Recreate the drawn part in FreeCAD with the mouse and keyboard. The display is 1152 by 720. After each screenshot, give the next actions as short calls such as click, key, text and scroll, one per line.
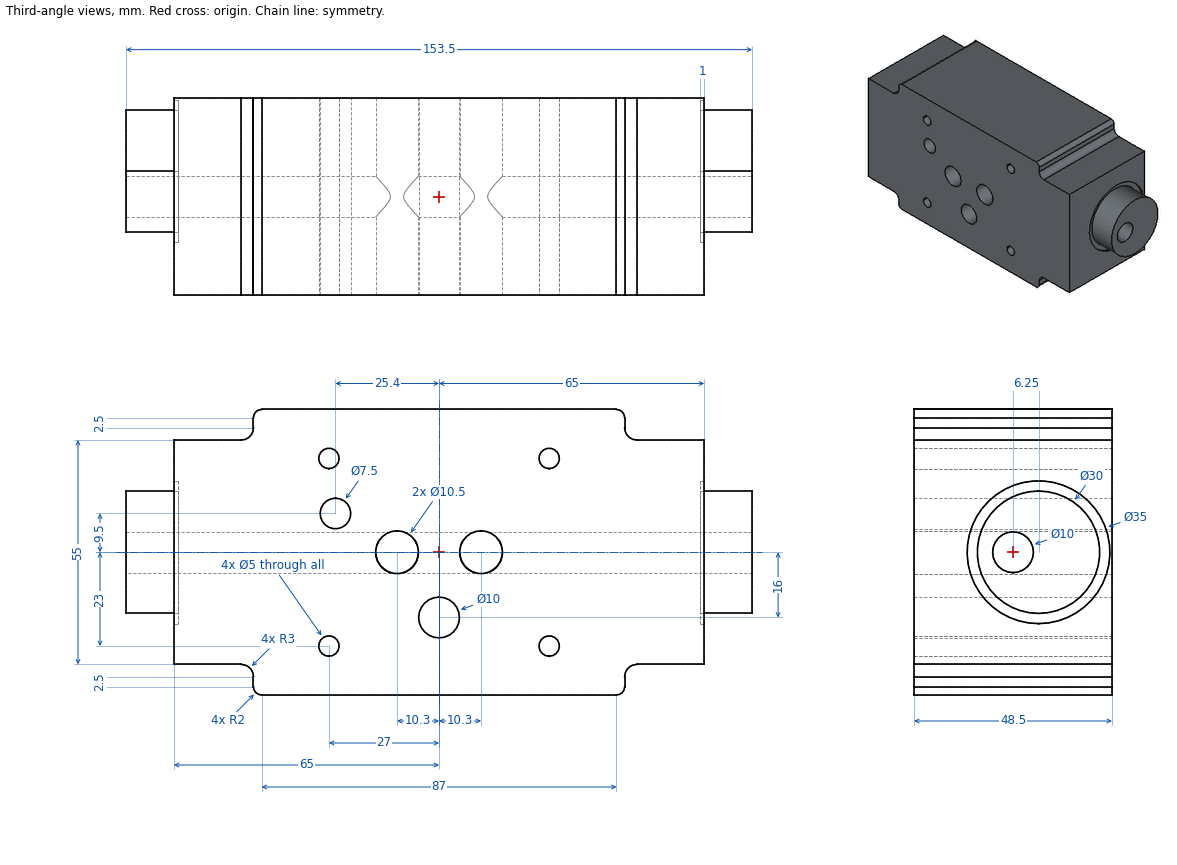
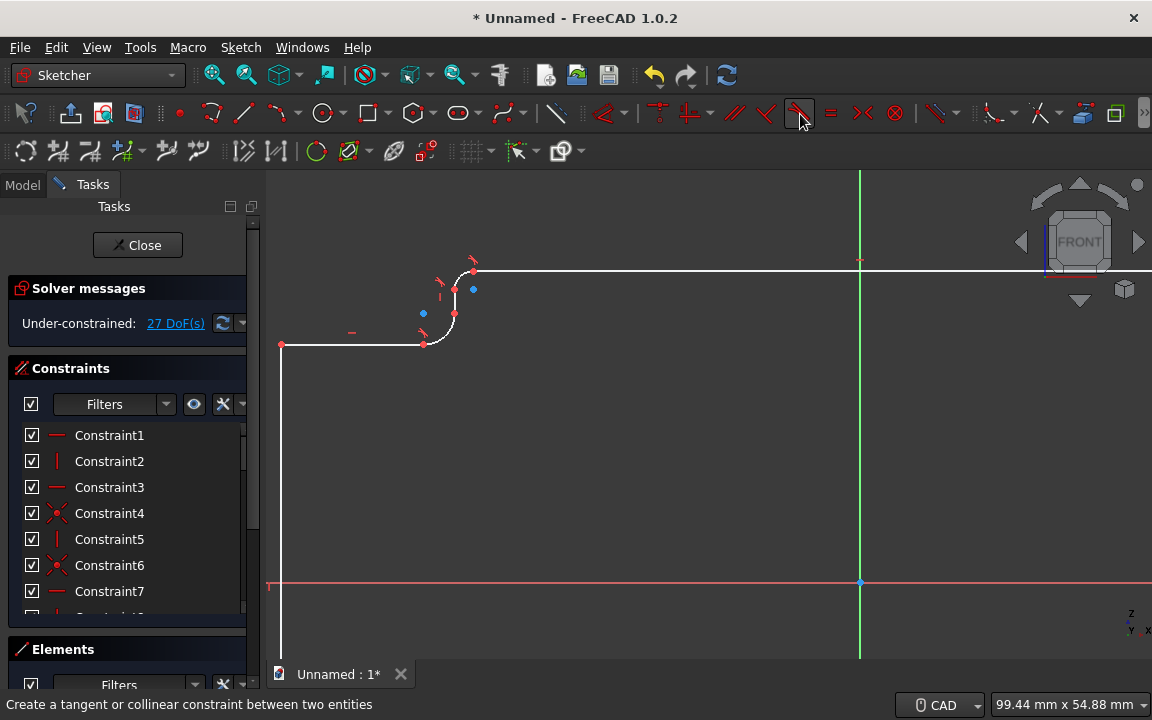
click(706, 271)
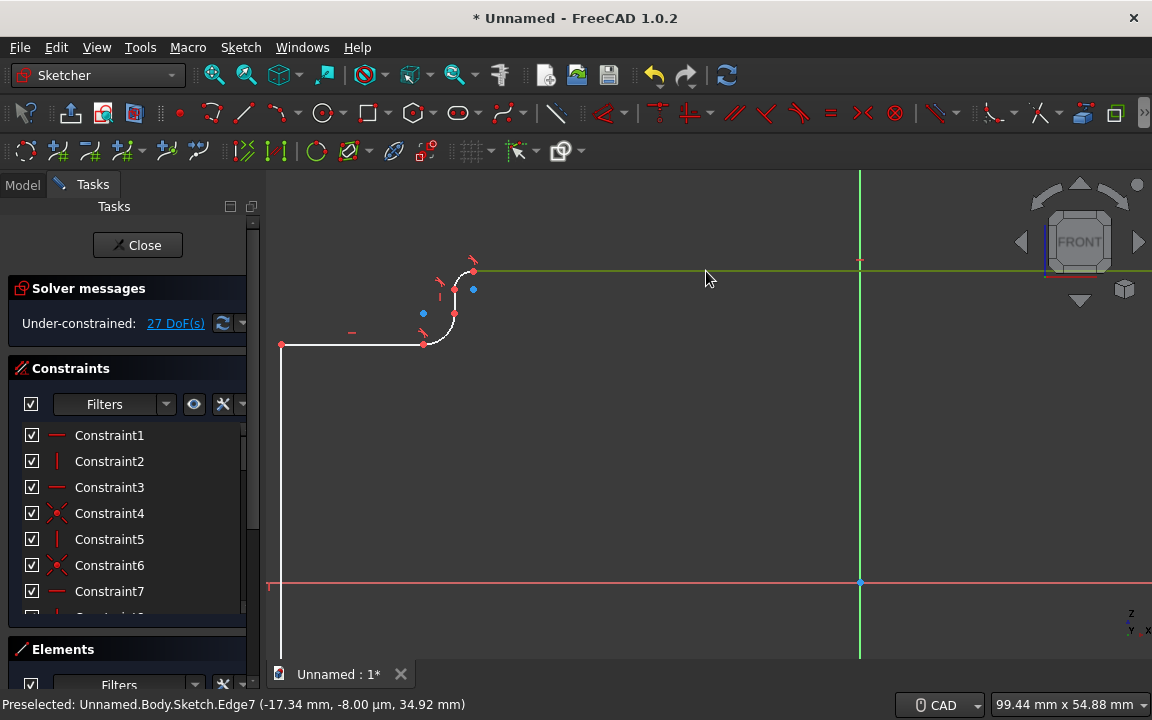
scroll(461, 277, down, 4)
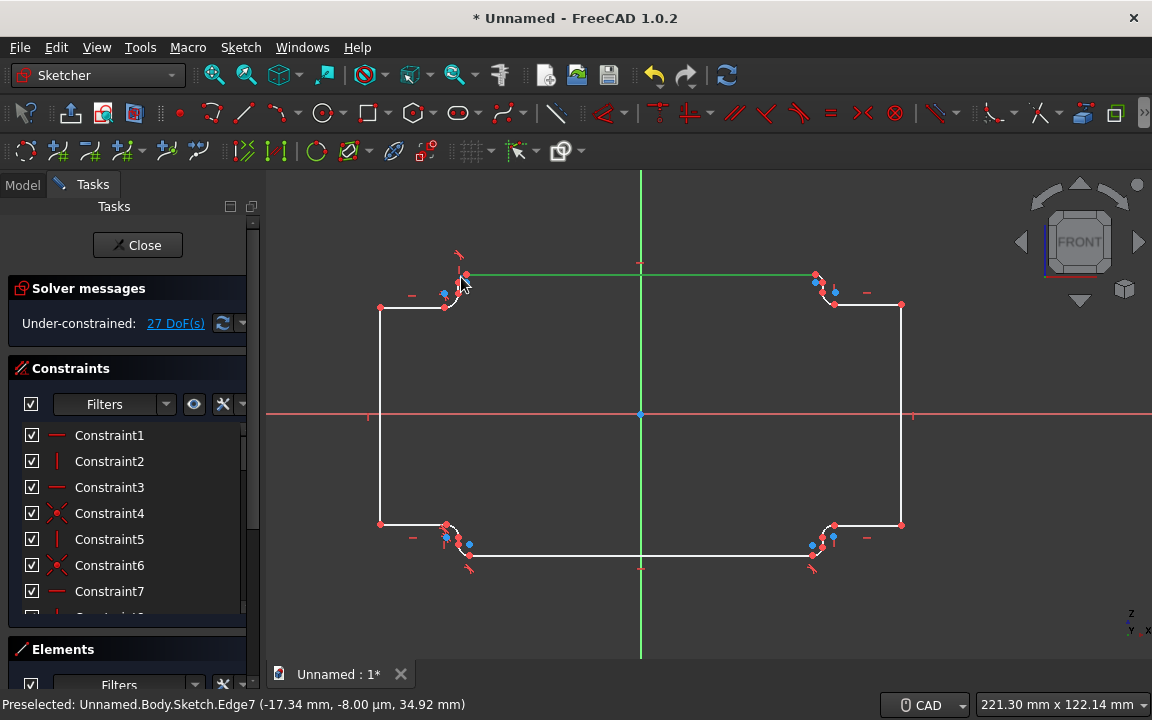
scroll(821, 277, up, 5)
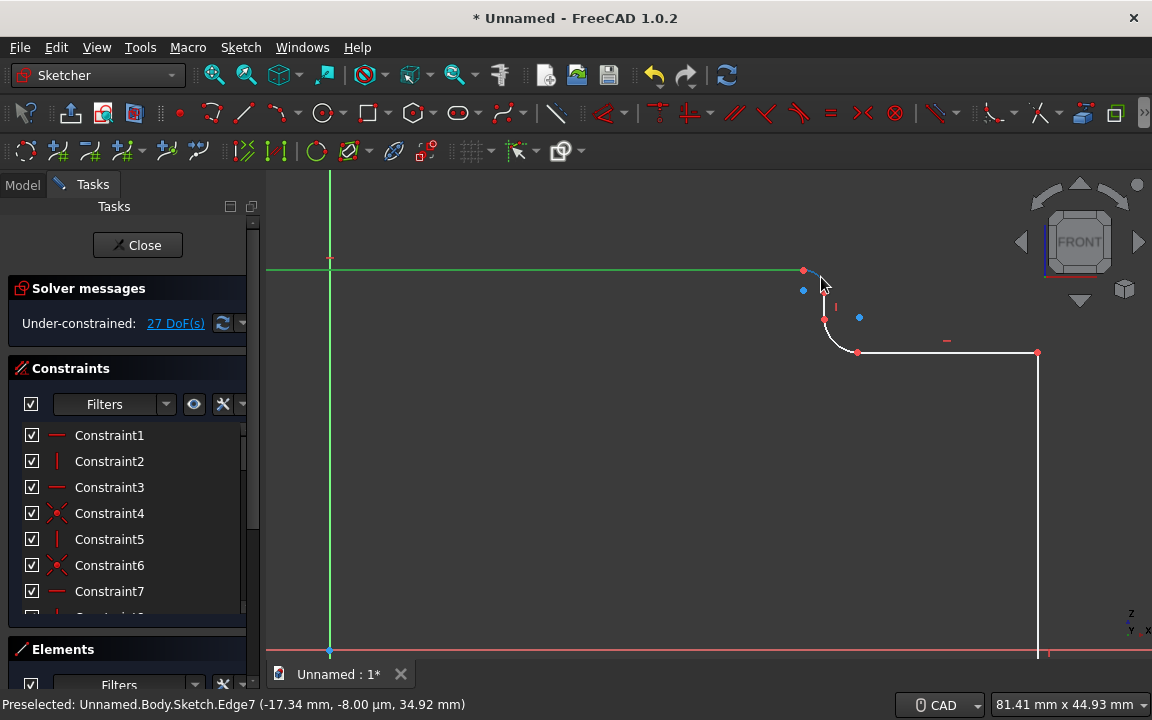
click(819, 277)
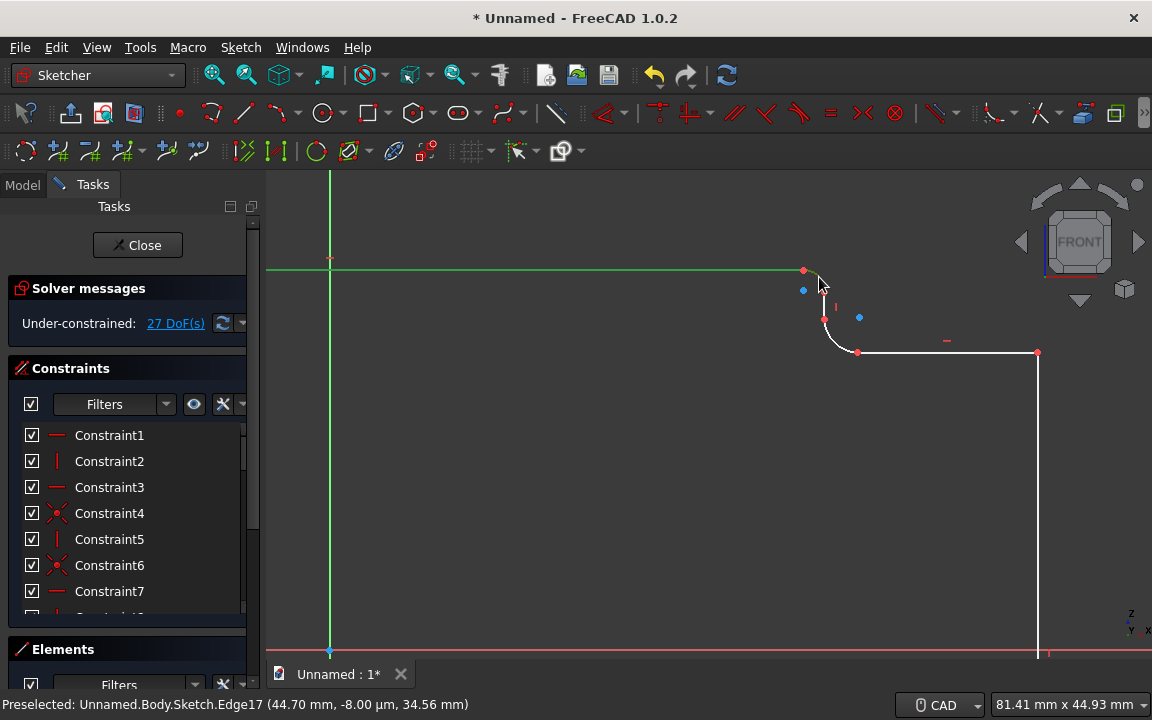
click(800, 114)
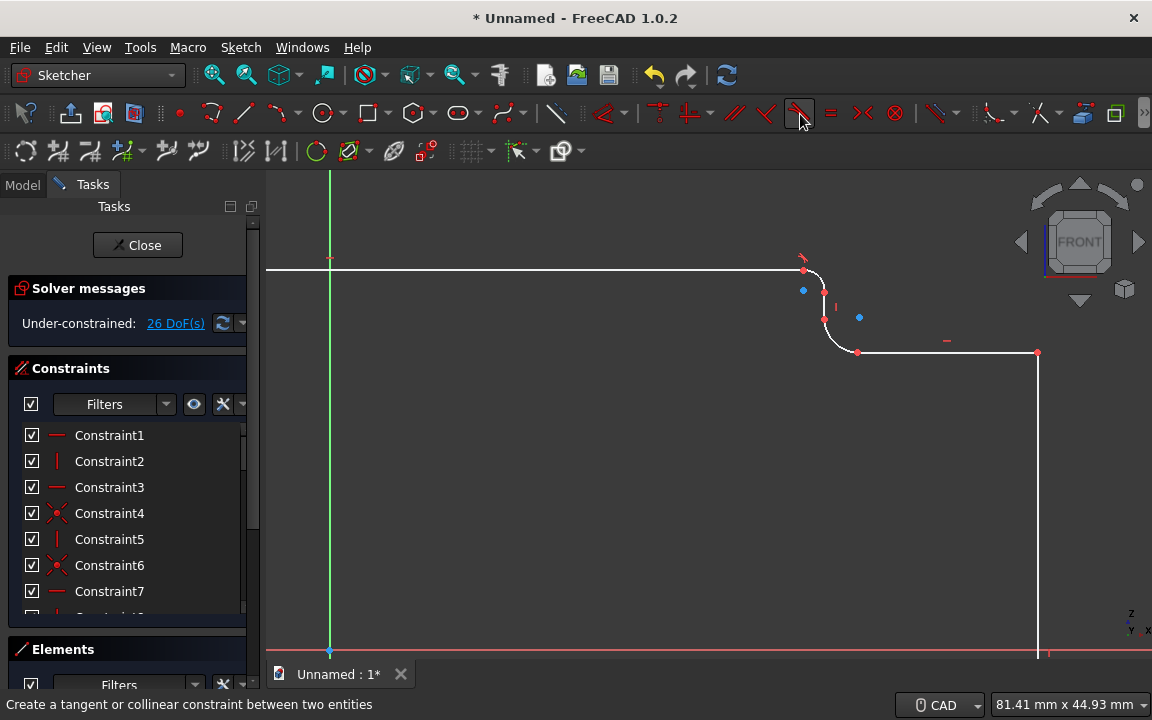
scroll(824, 303, up, 2)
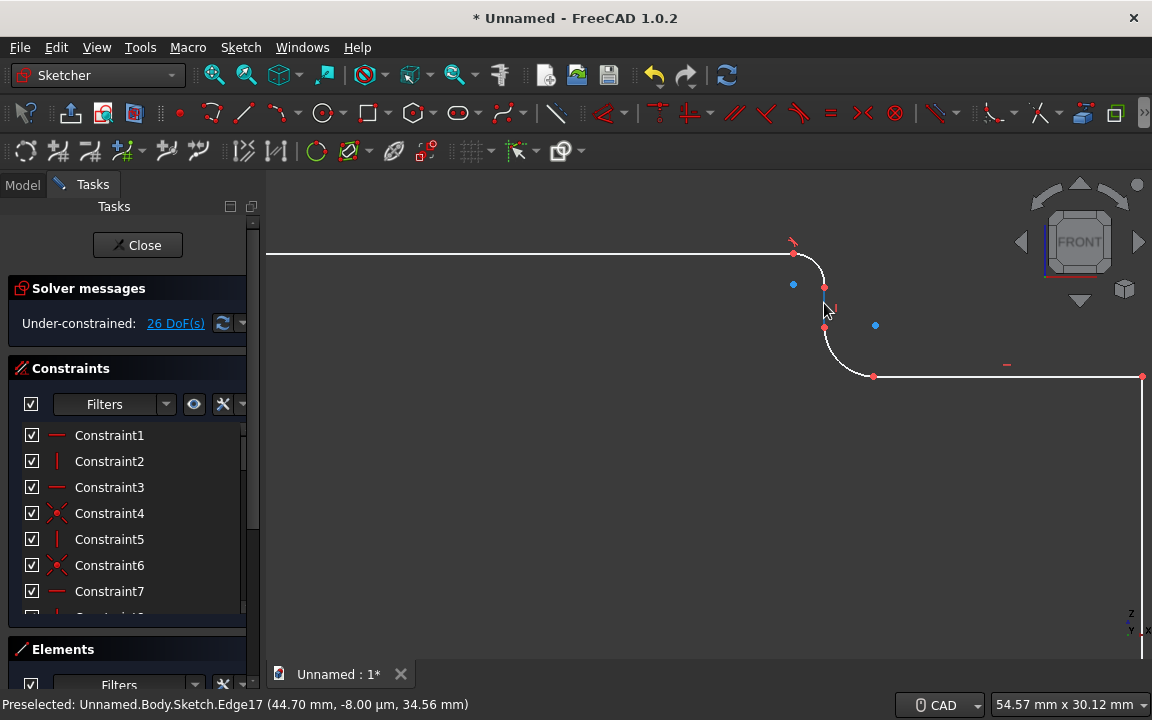
click(824, 303)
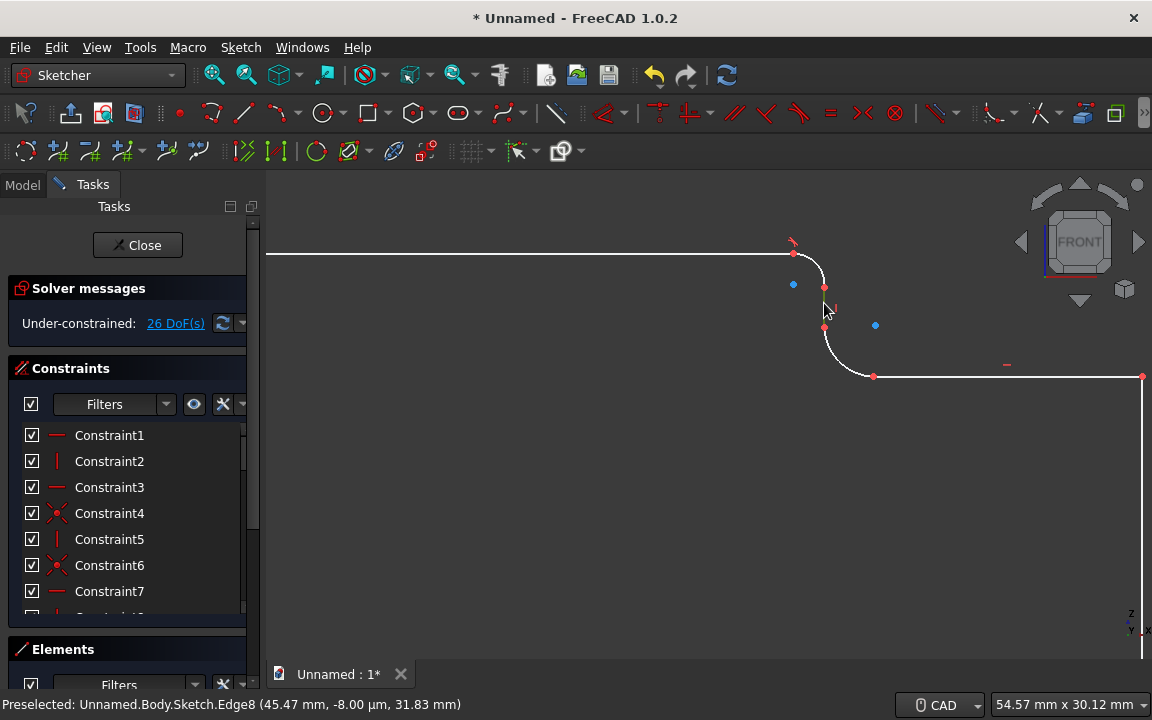
click(822, 272)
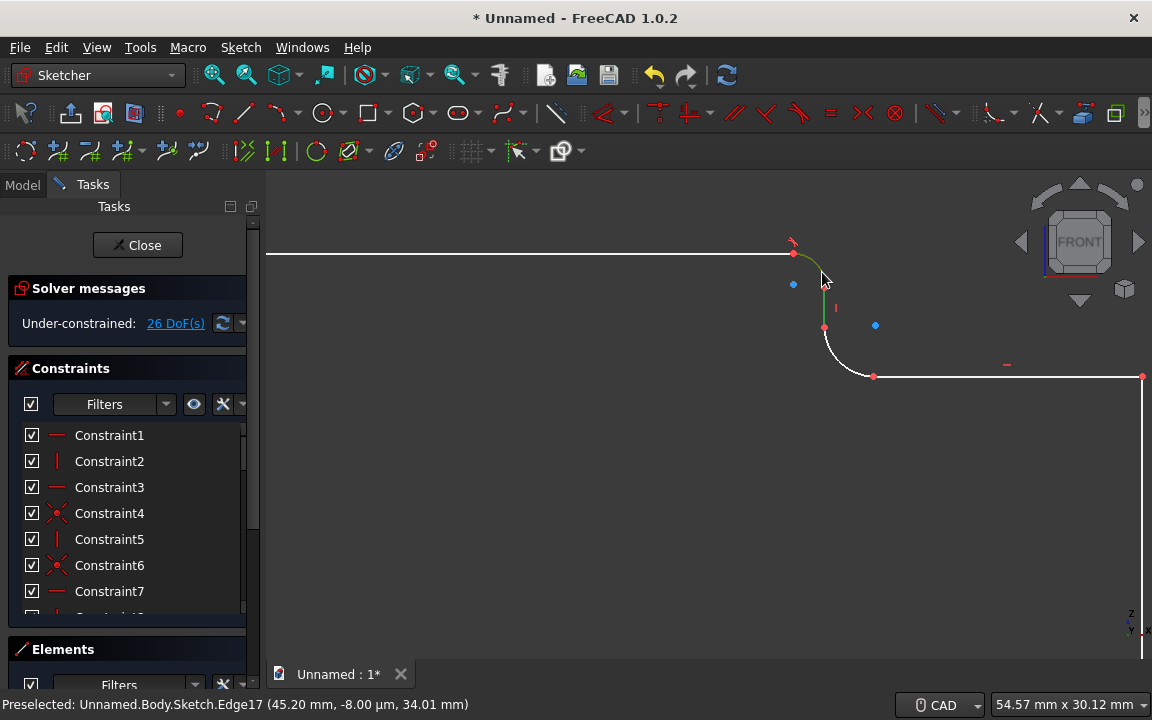
click(800, 114)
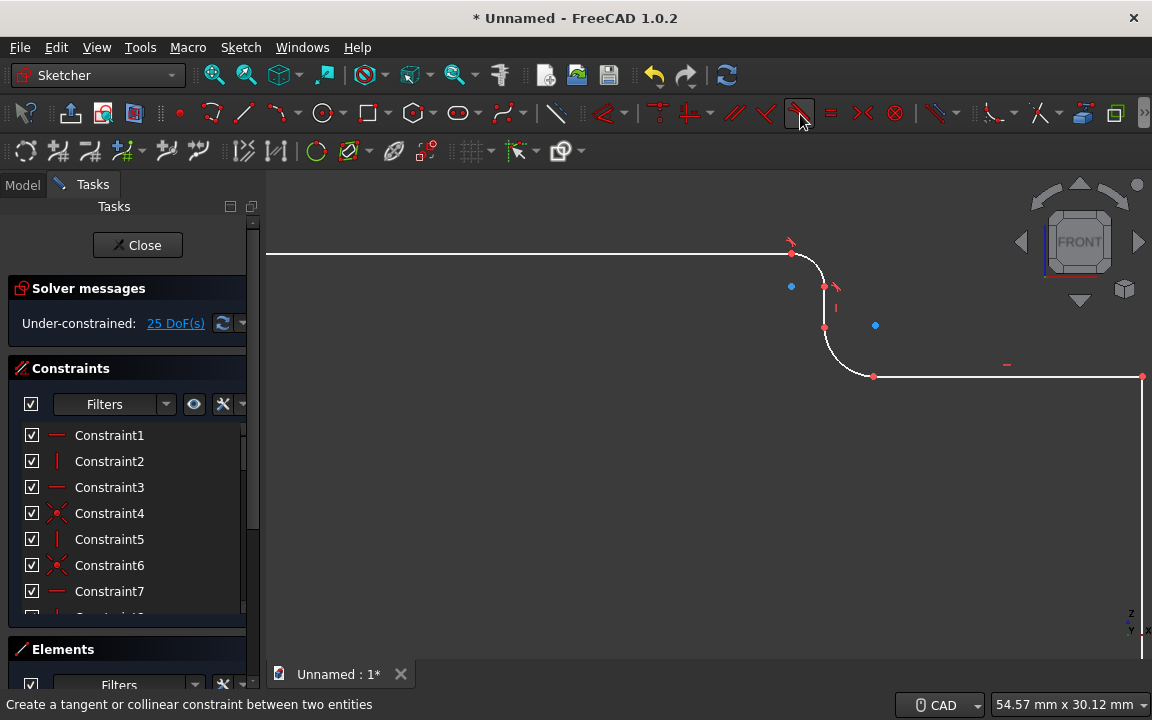
click(824, 299)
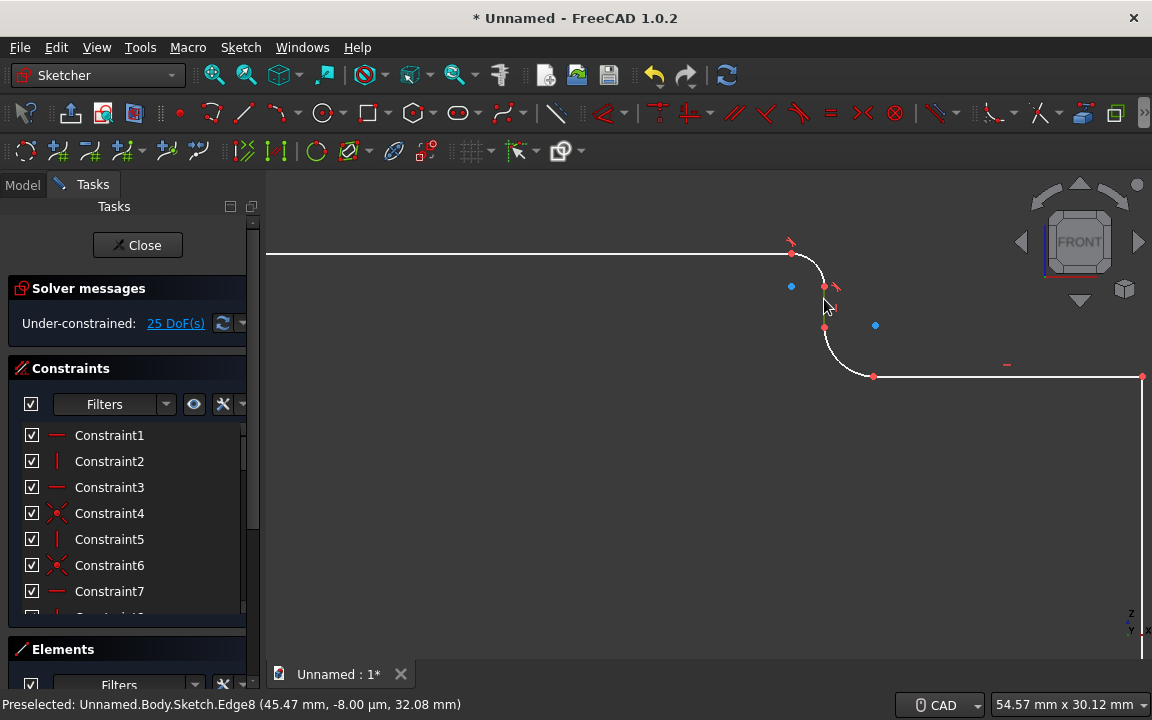
click(830, 350)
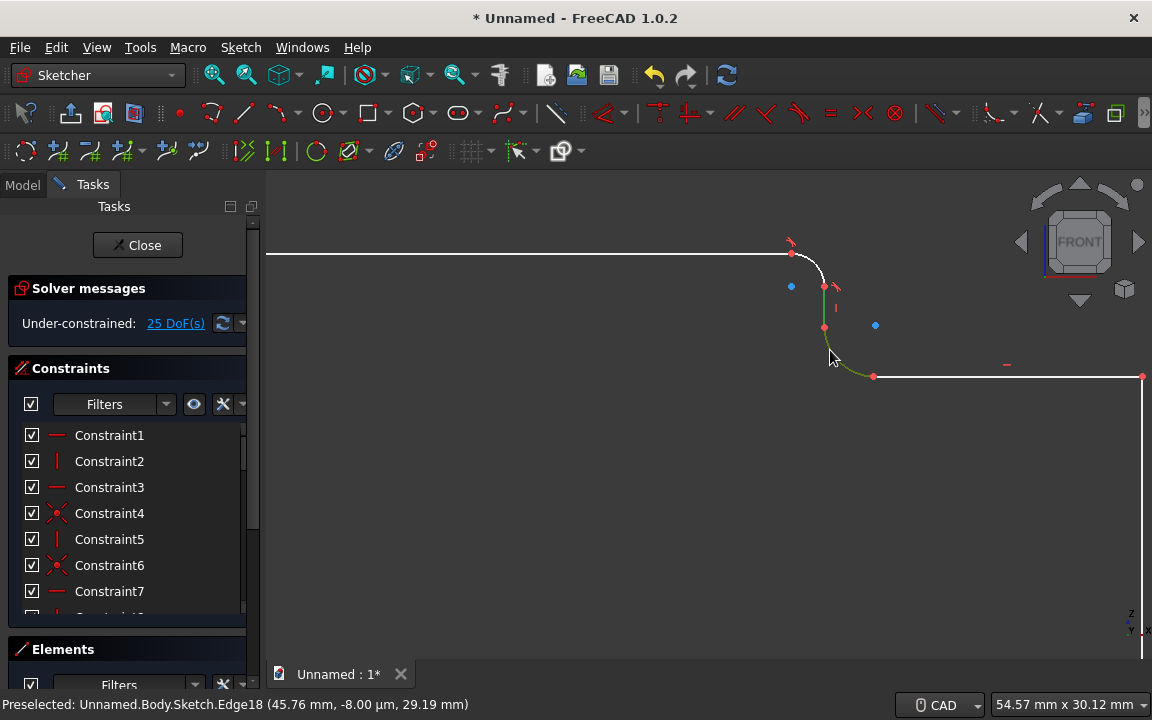
click(800, 114)